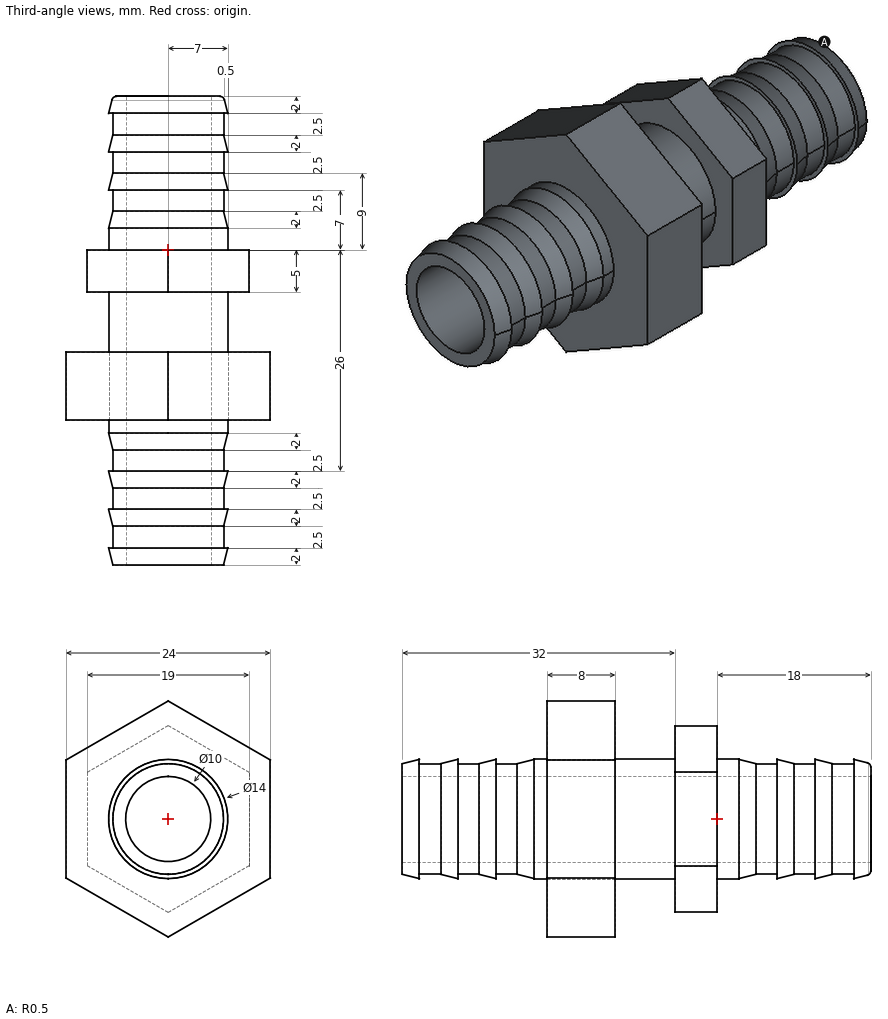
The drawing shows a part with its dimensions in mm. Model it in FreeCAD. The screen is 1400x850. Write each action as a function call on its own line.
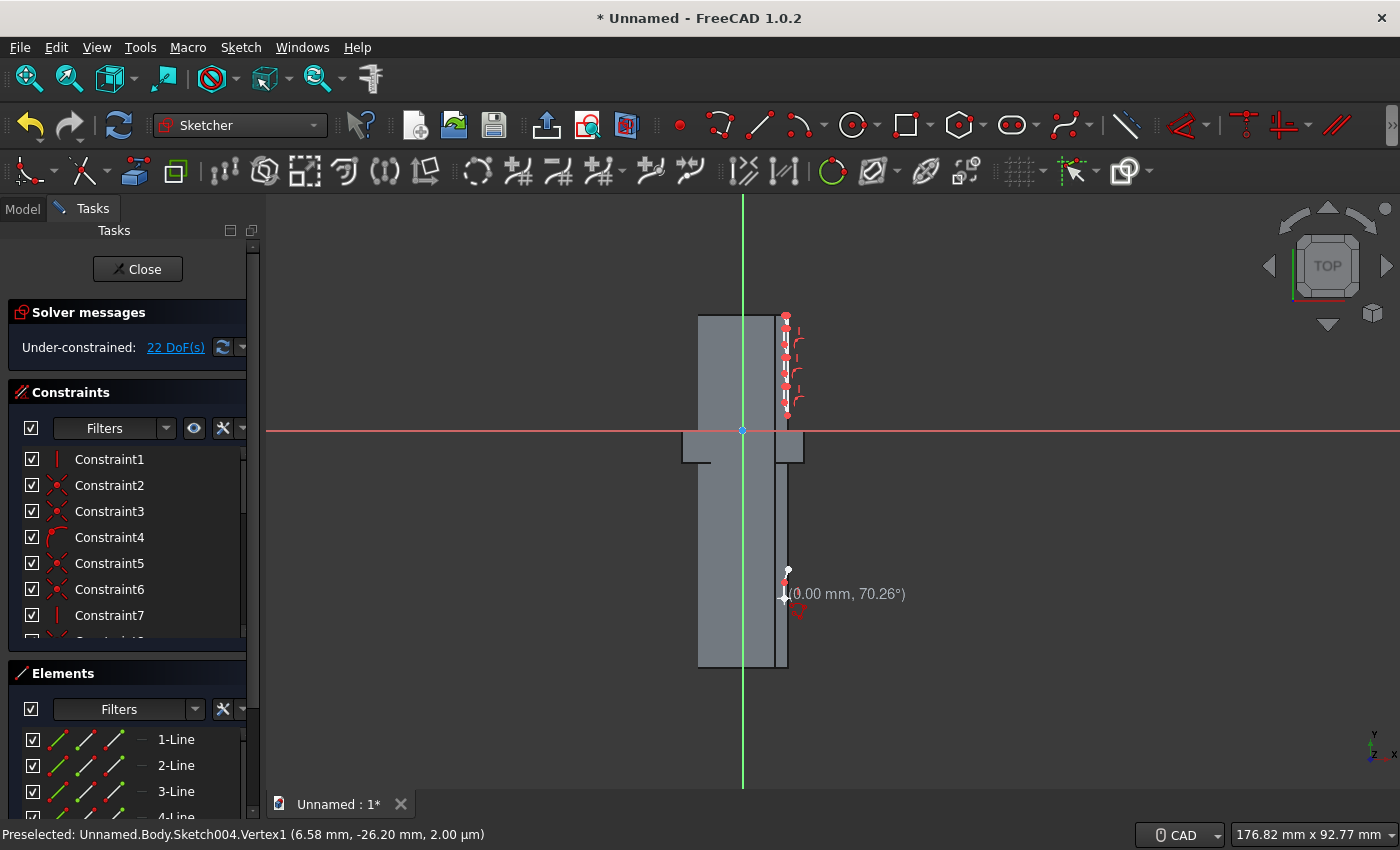
scroll(788, 598, up, 8)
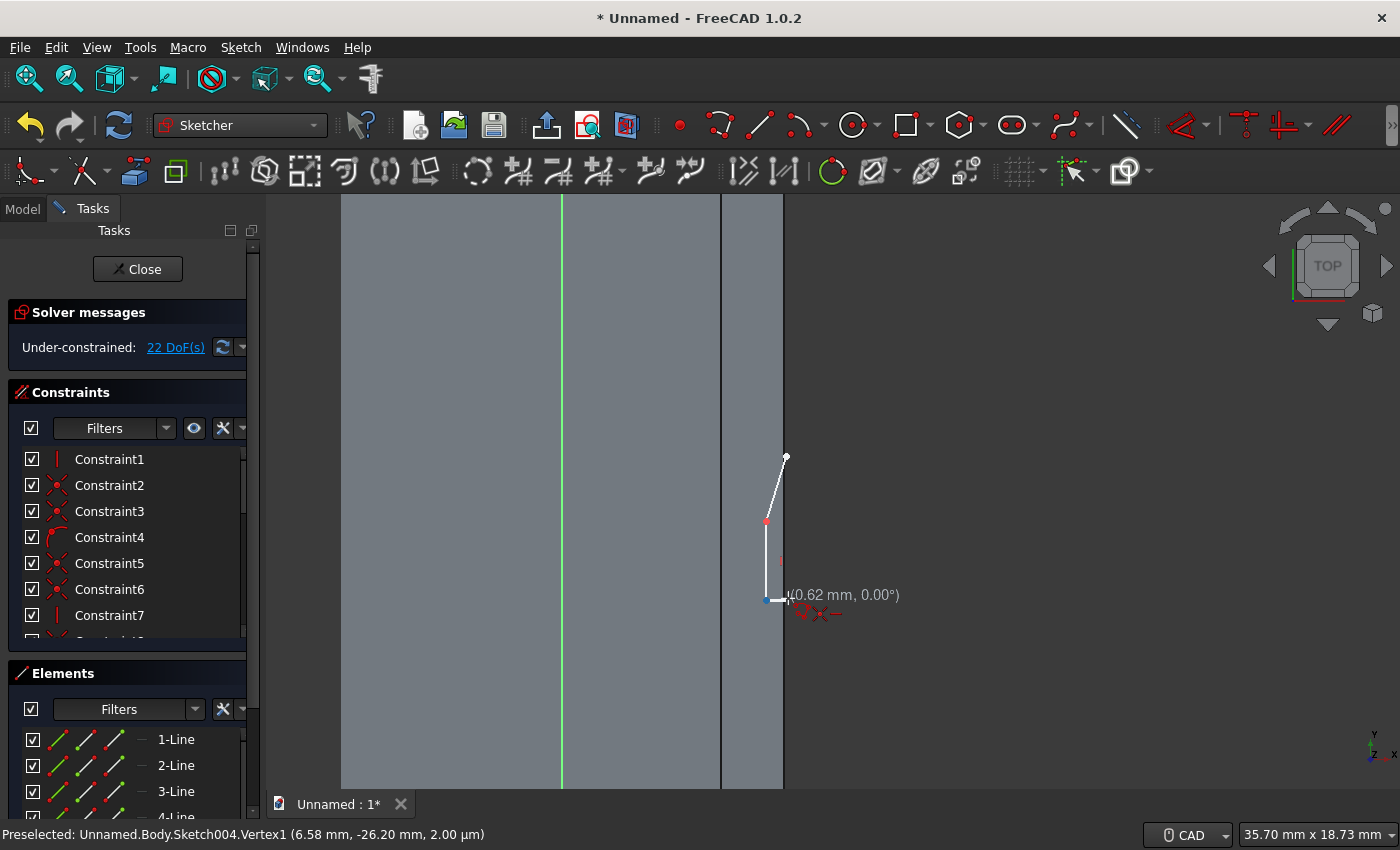
click(784, 595)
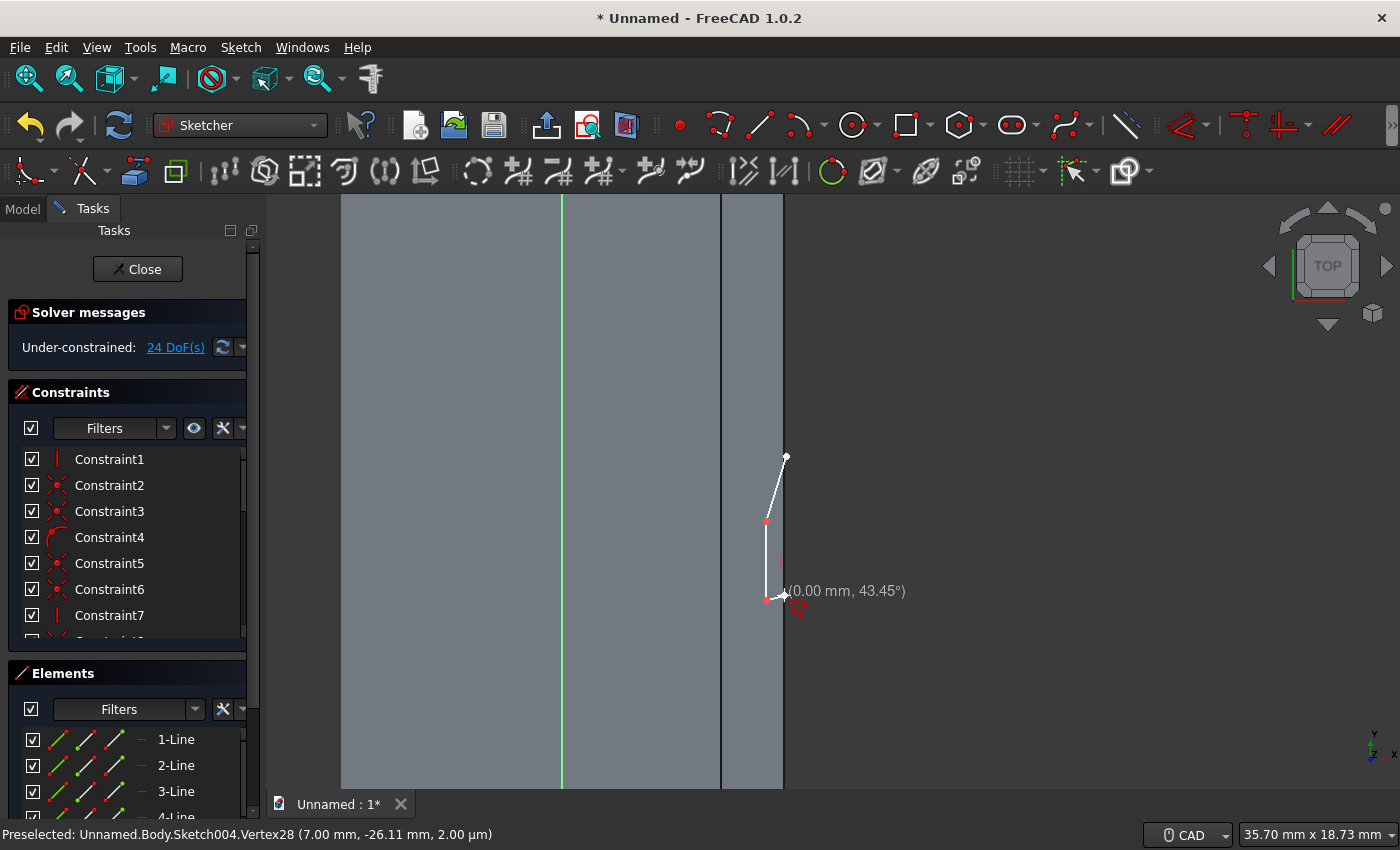
scroll(788, 598, down, 8)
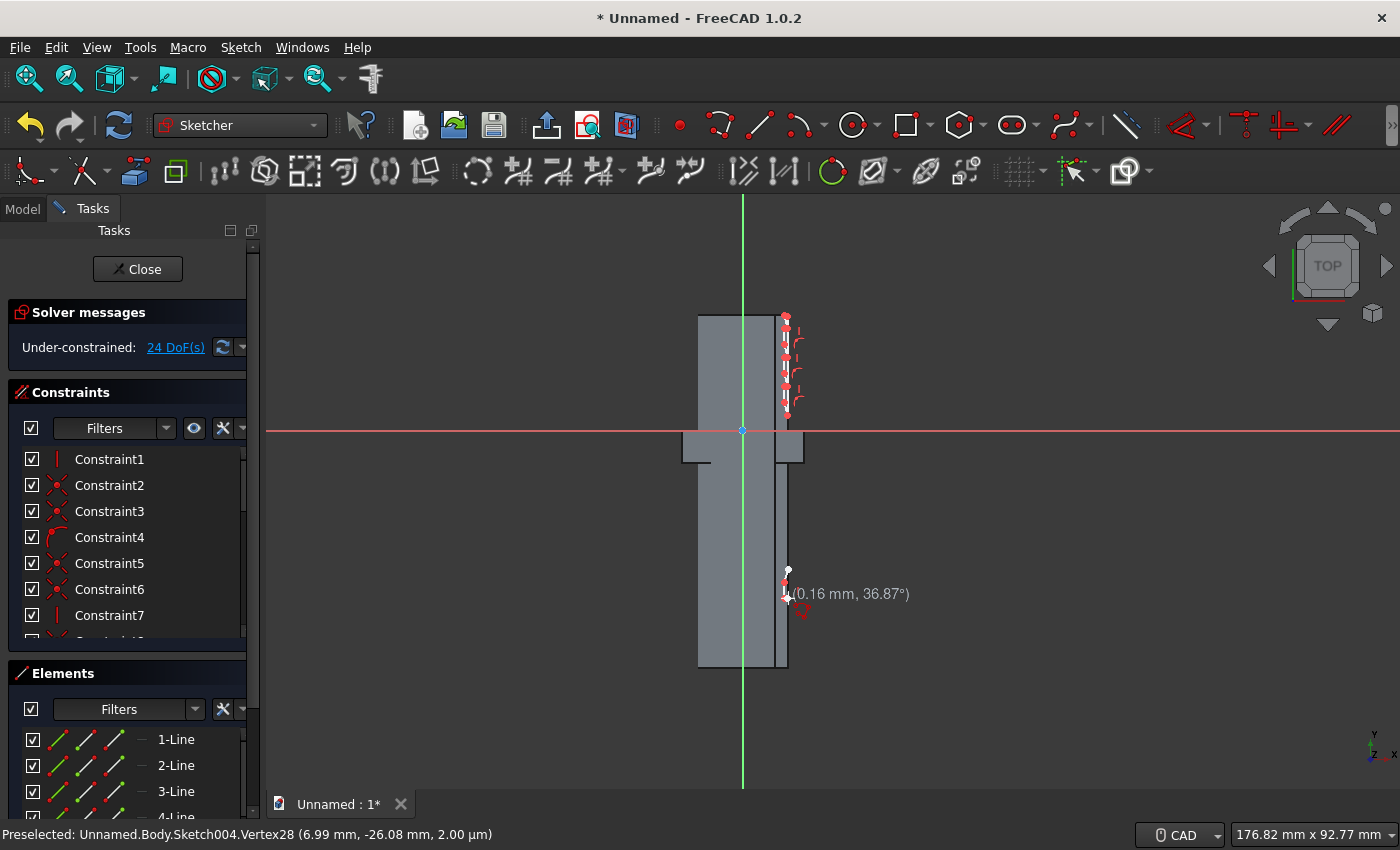
scroll(784, 610, up, 2)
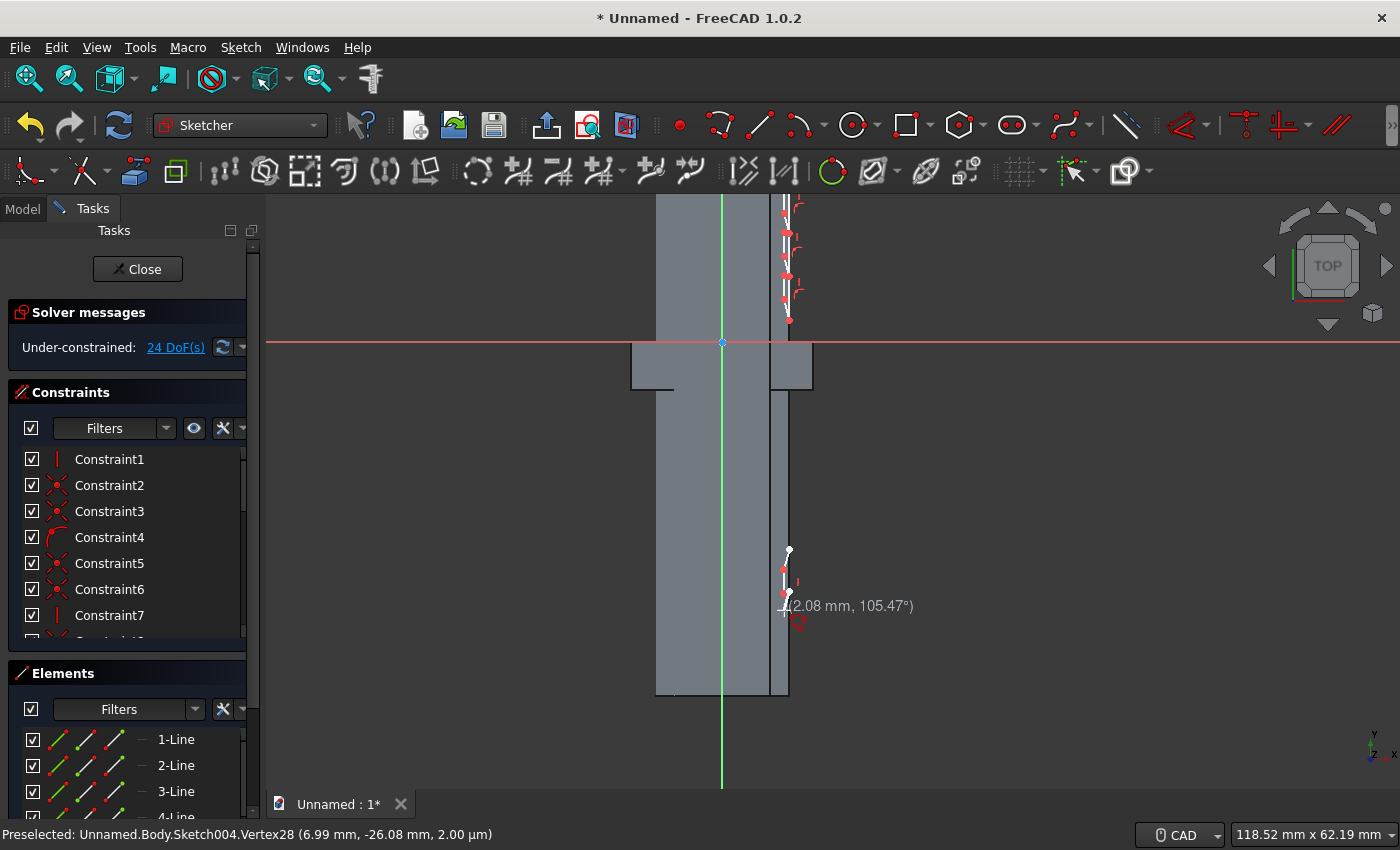
click(784, 610)
click(784, 634)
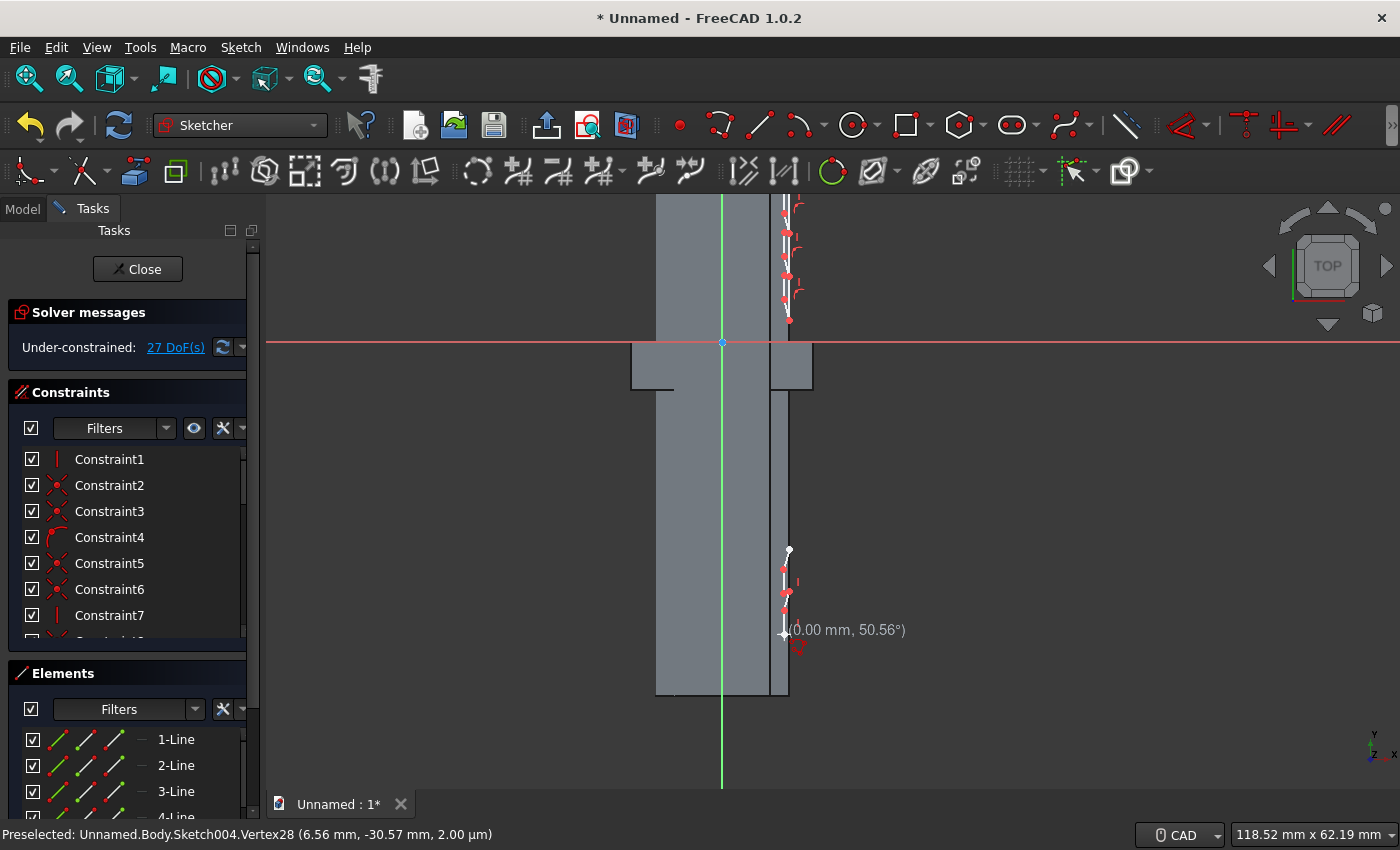
scroll(789, 634, up, 6)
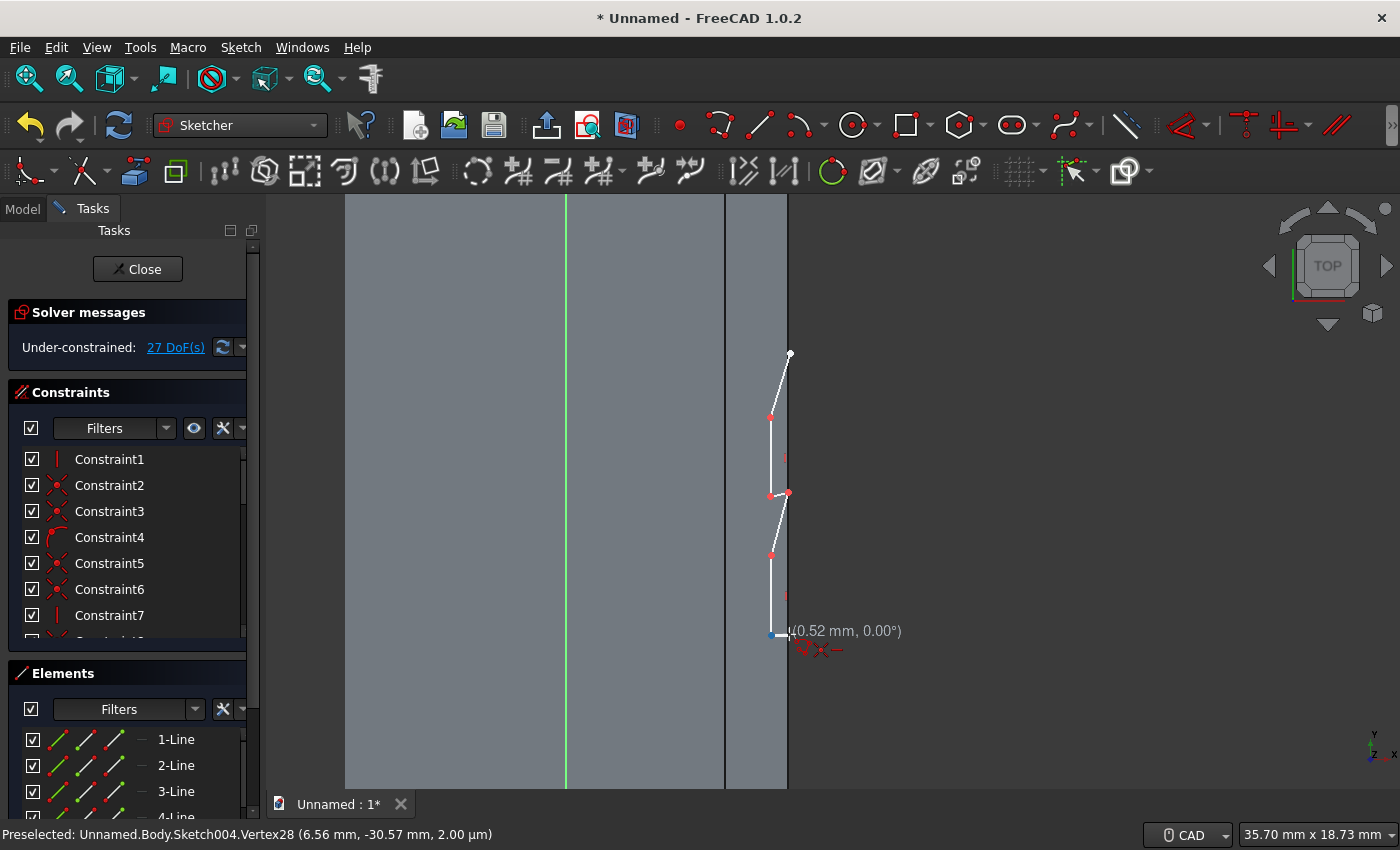
click(788, 632)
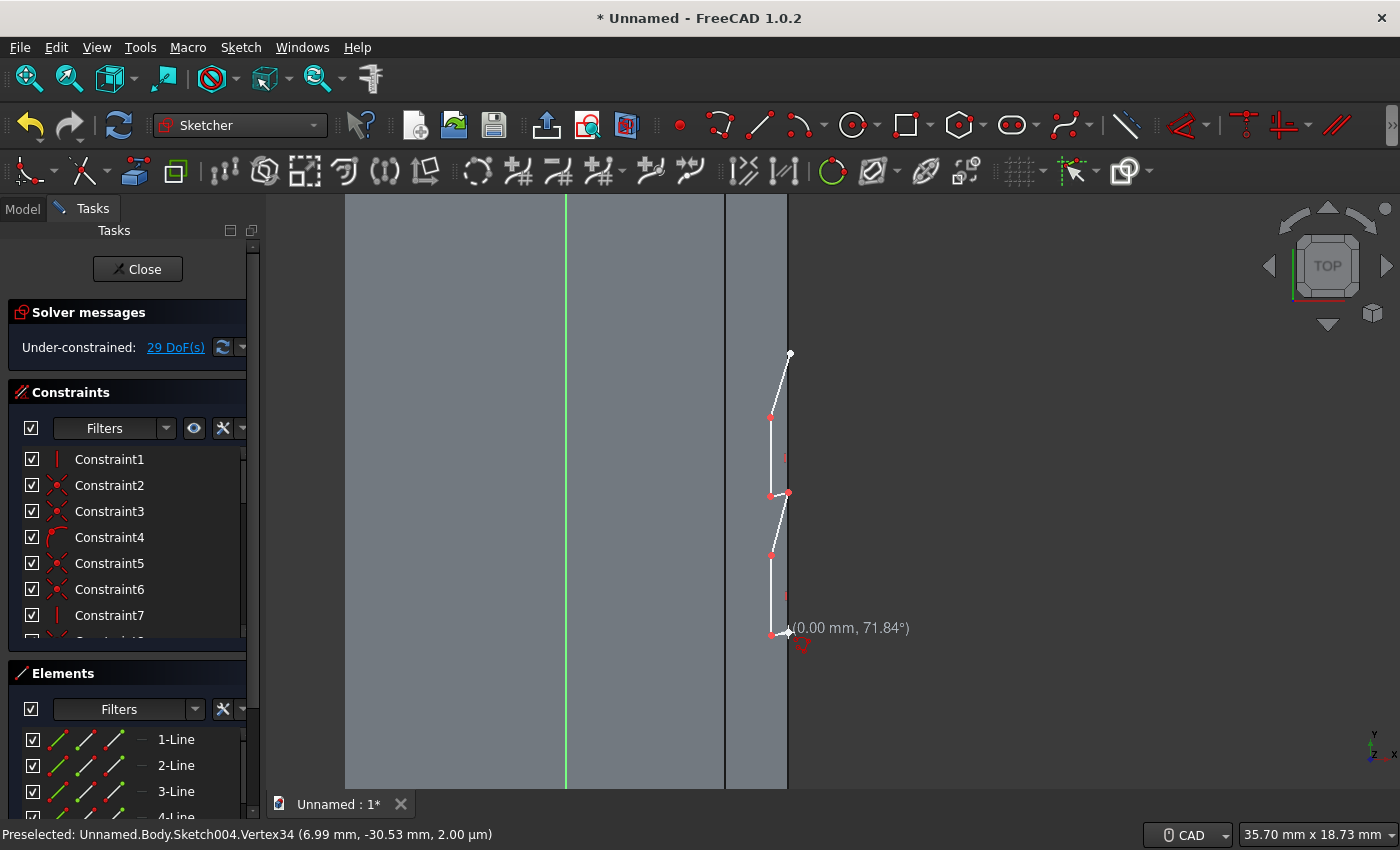
scroll(787, 624, down, 8)